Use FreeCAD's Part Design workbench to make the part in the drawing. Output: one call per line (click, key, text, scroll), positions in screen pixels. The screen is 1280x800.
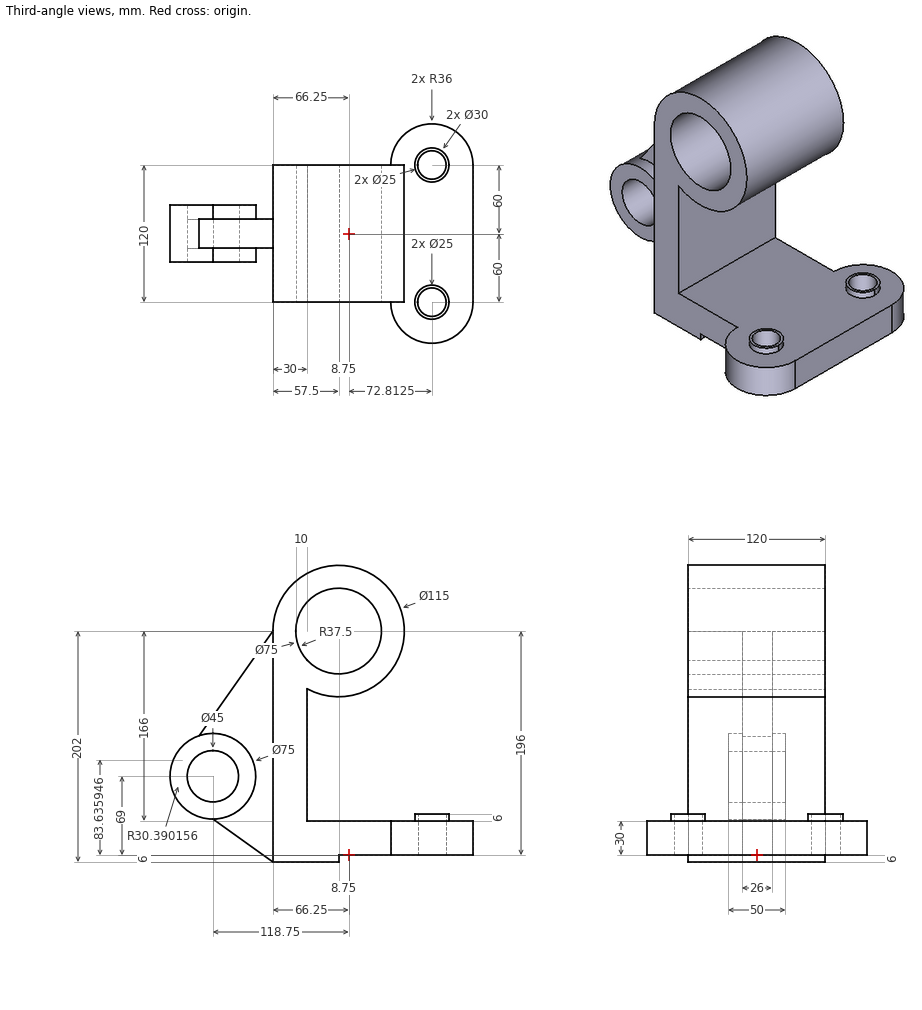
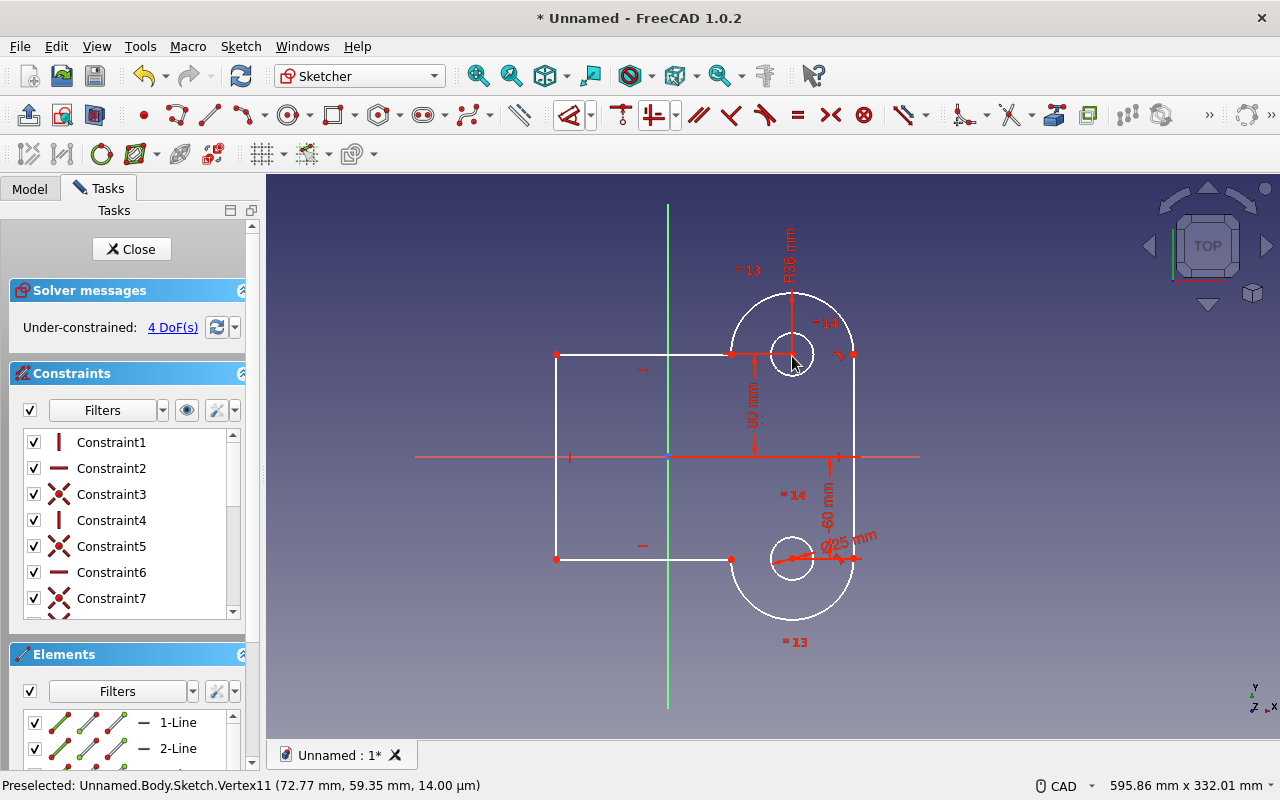
click(556, 416)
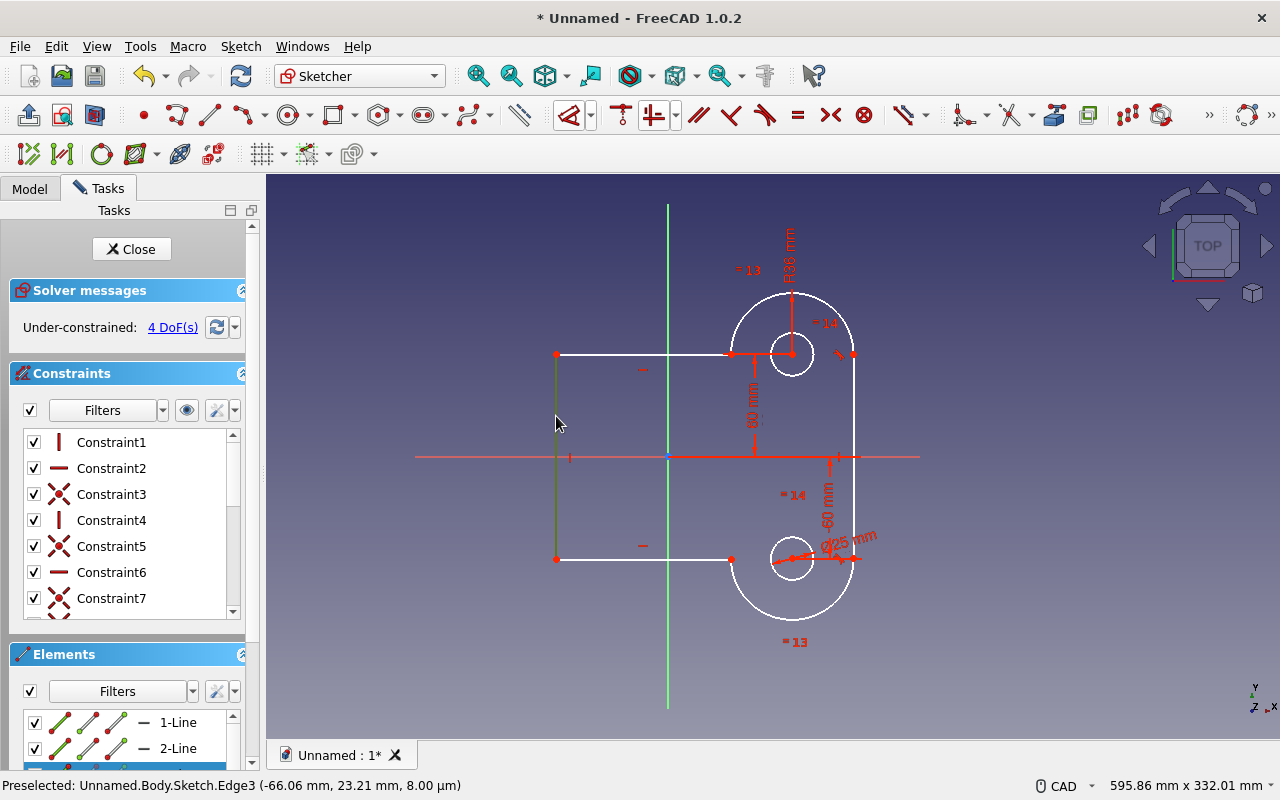
key(i)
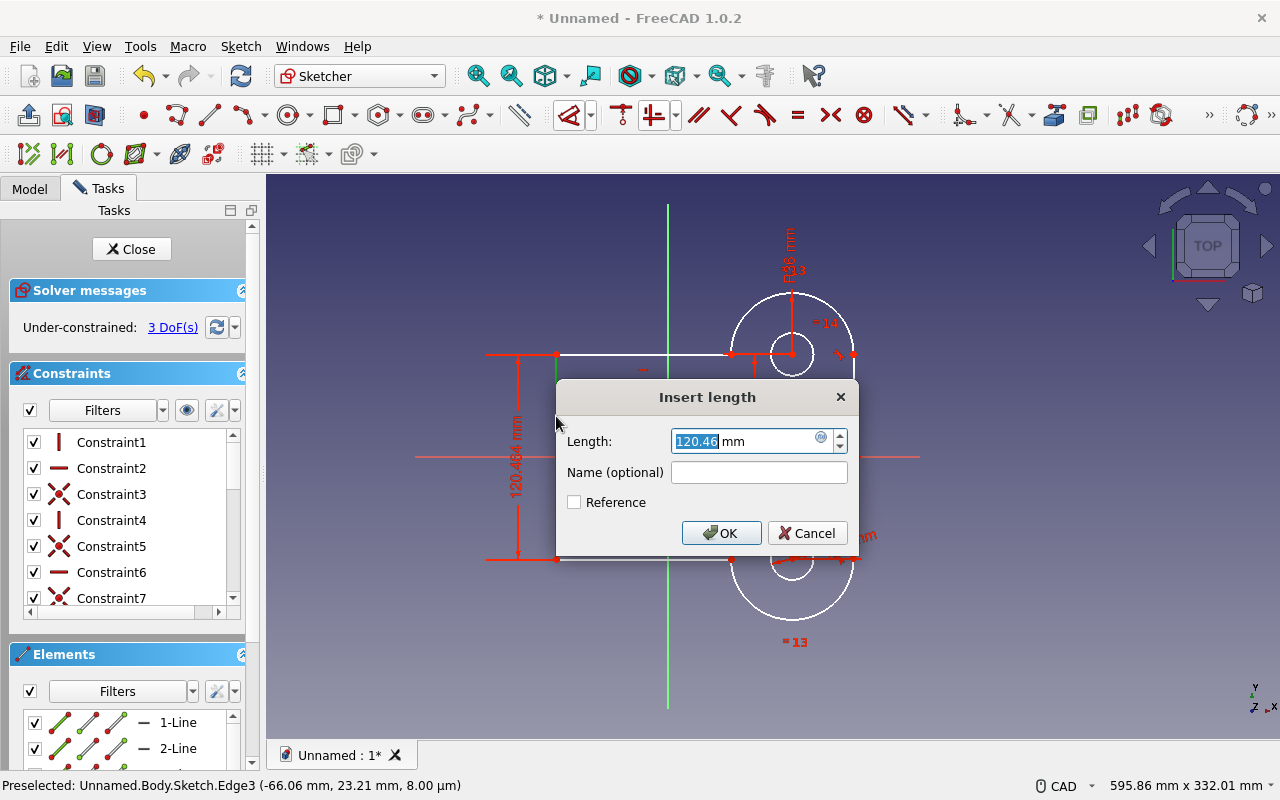
text(120)
key(Return)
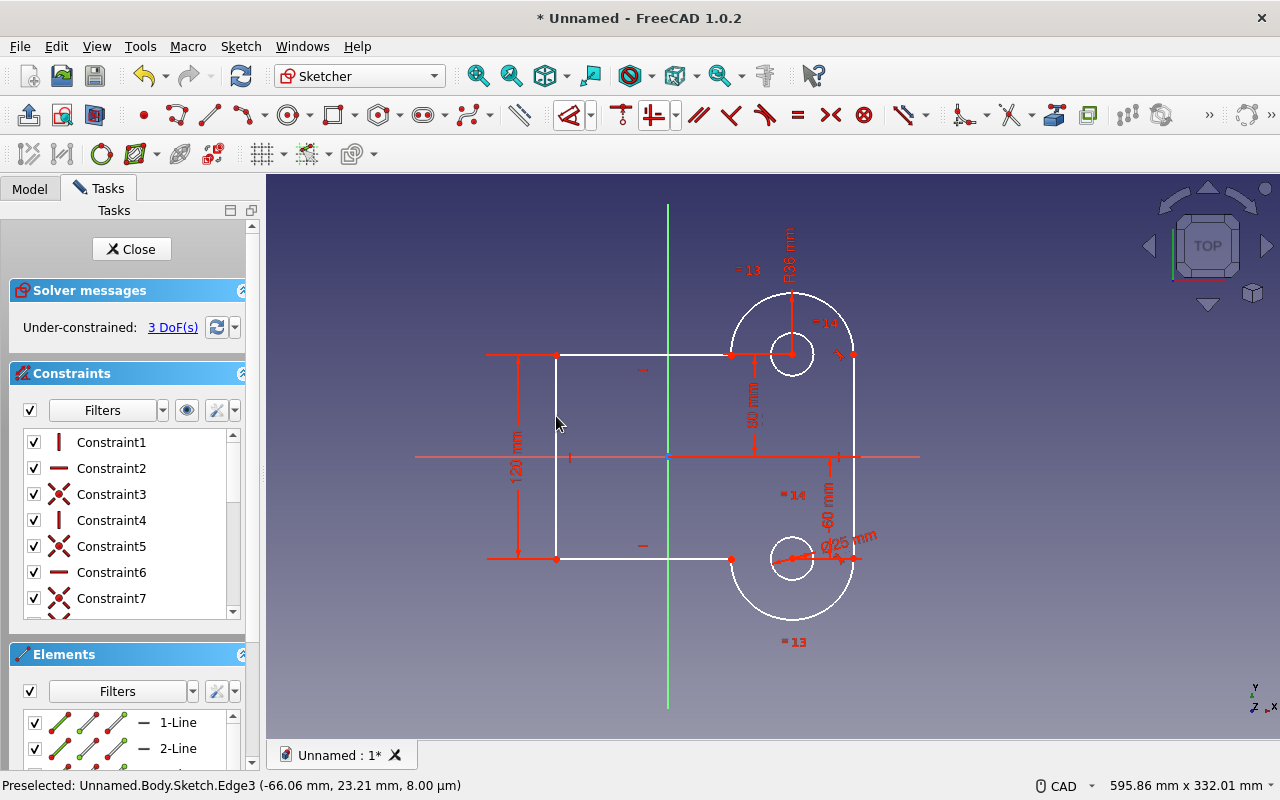
click(731, 355)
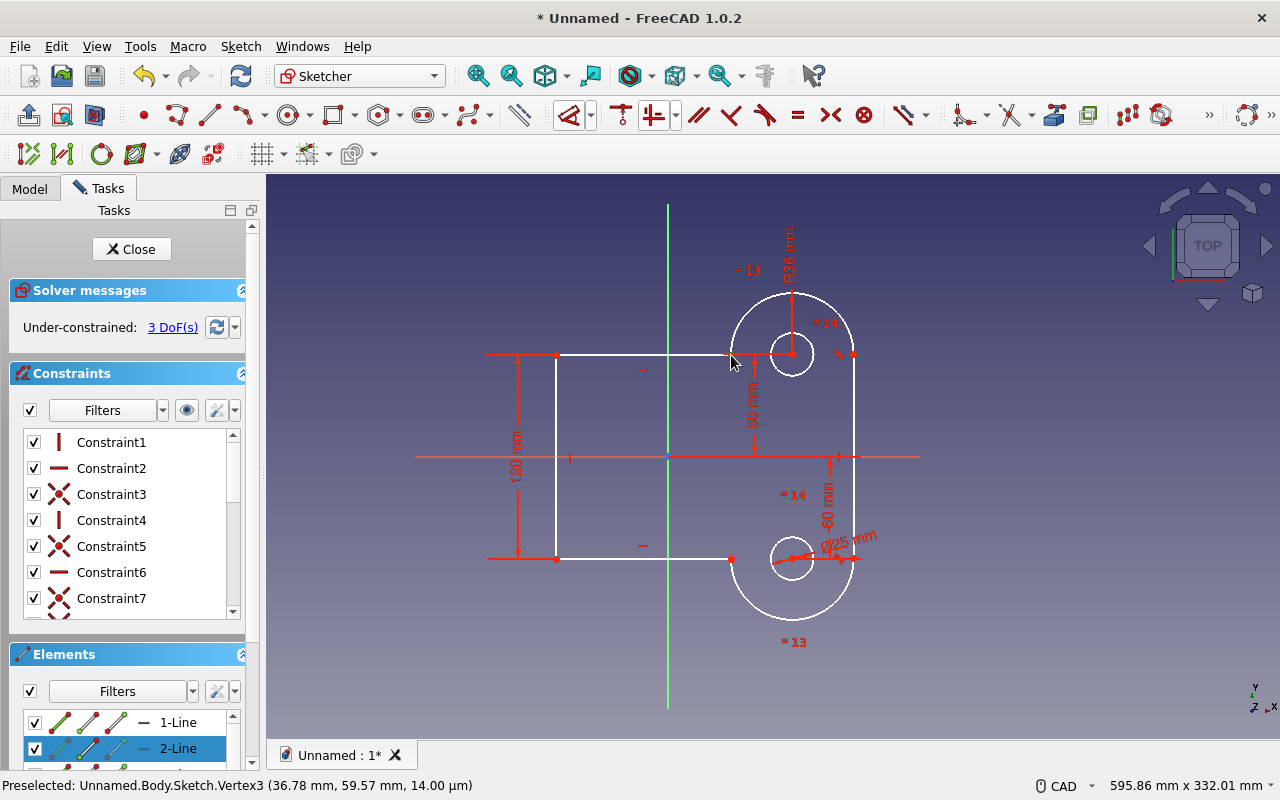
key(i)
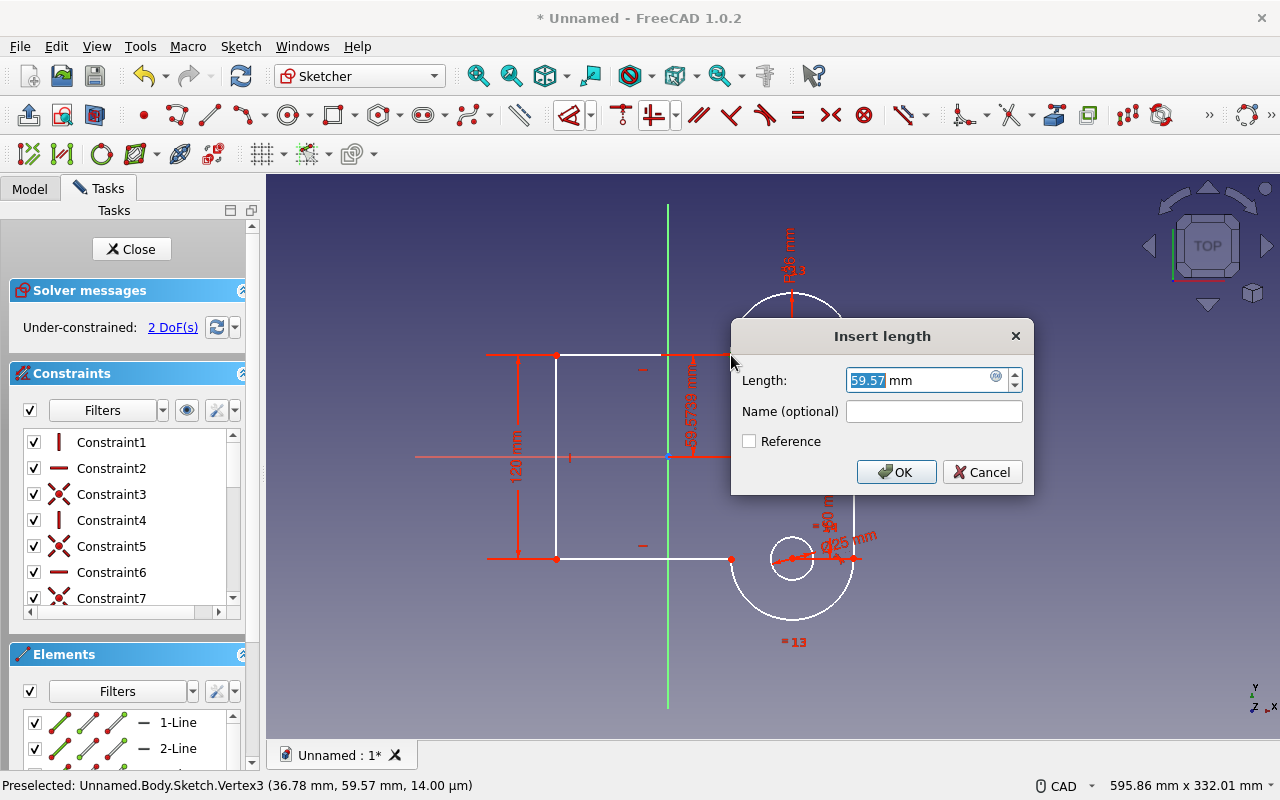
text(60)
key(Return)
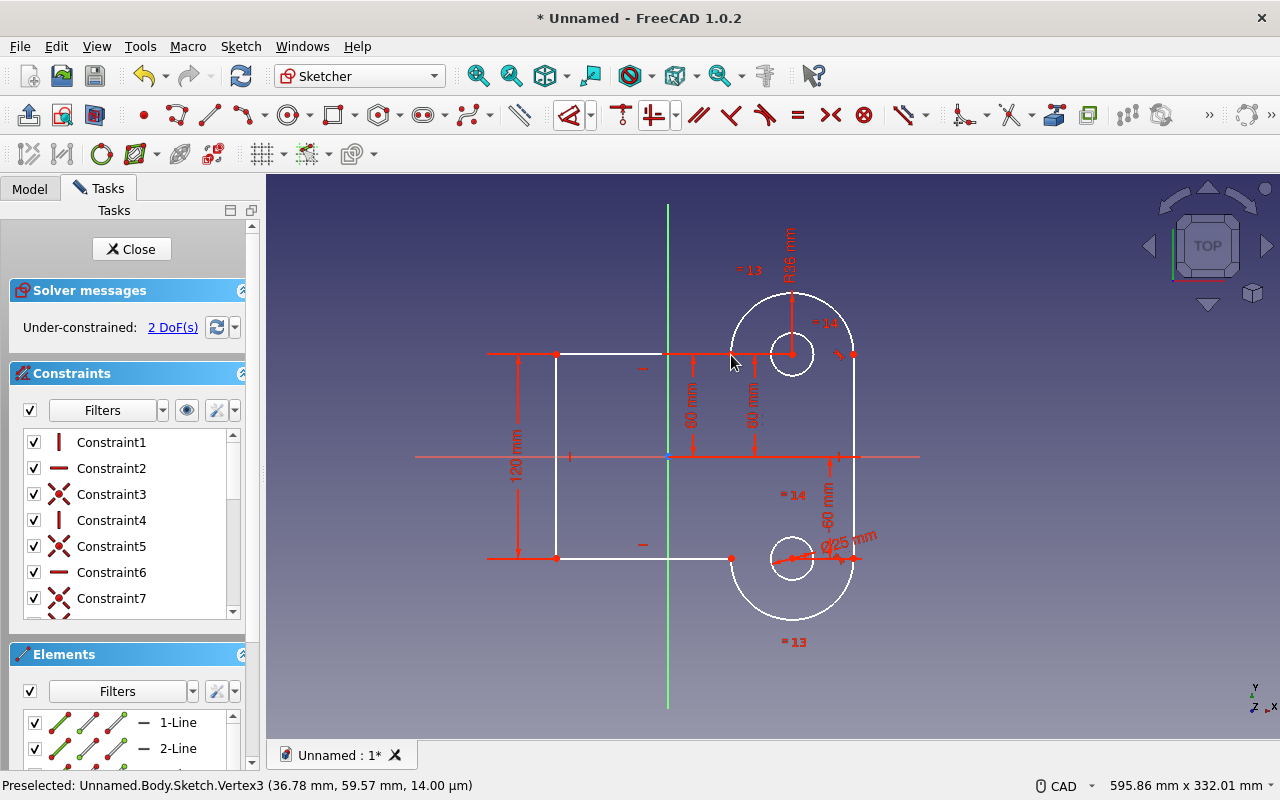
click(556, 354)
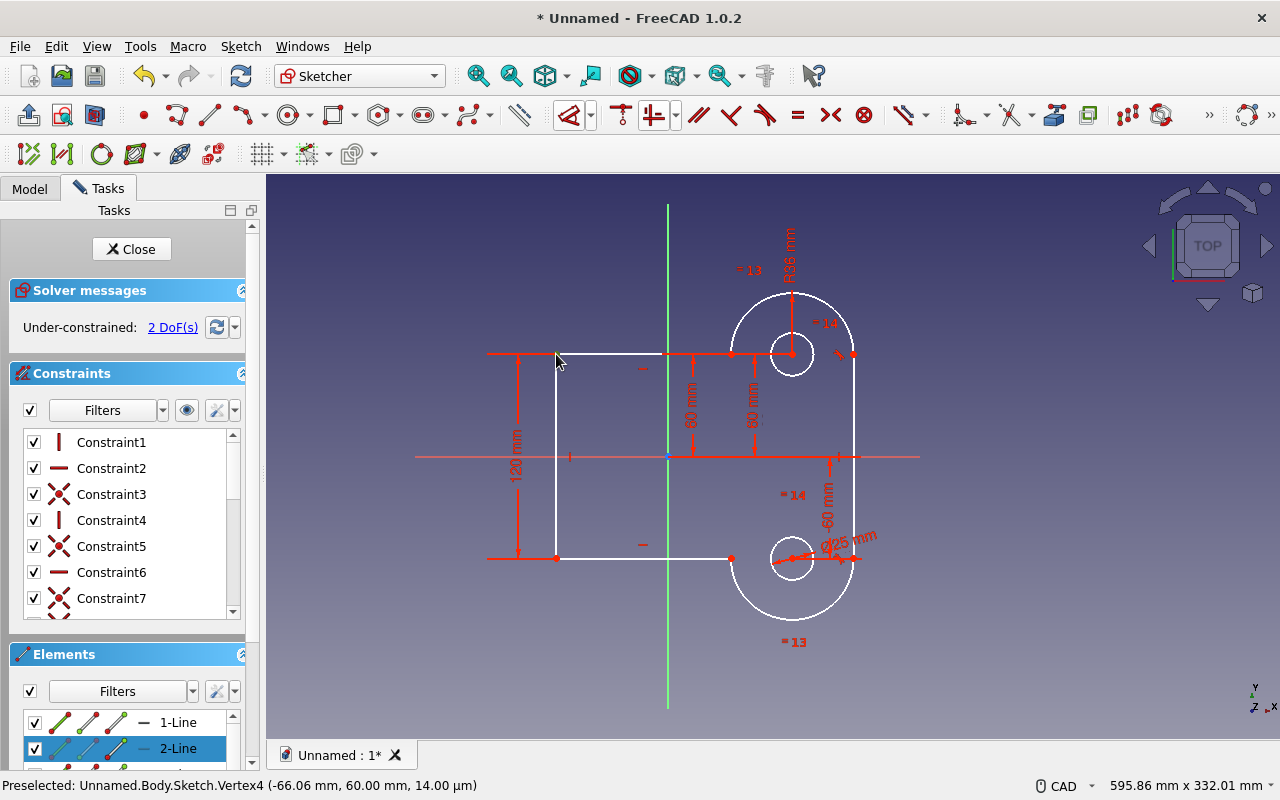
key(l)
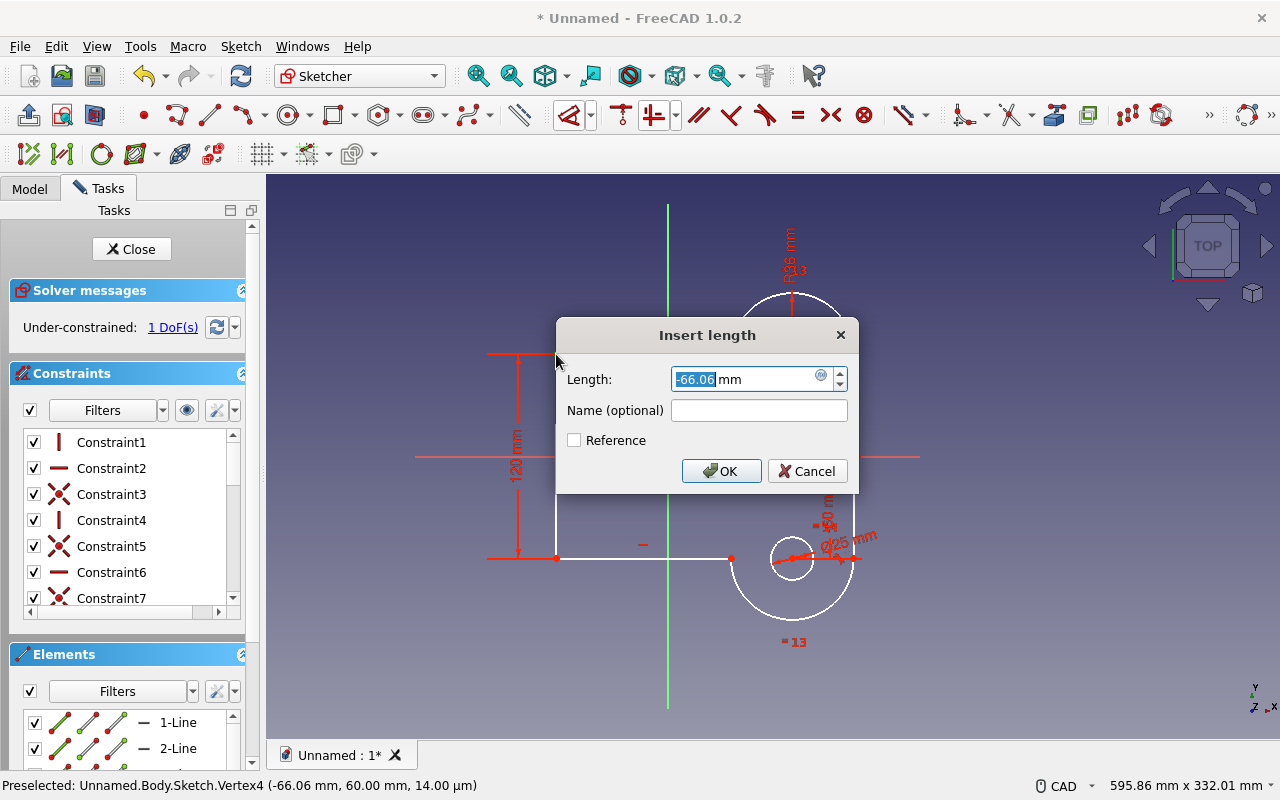
text(-66.25)
key(Return)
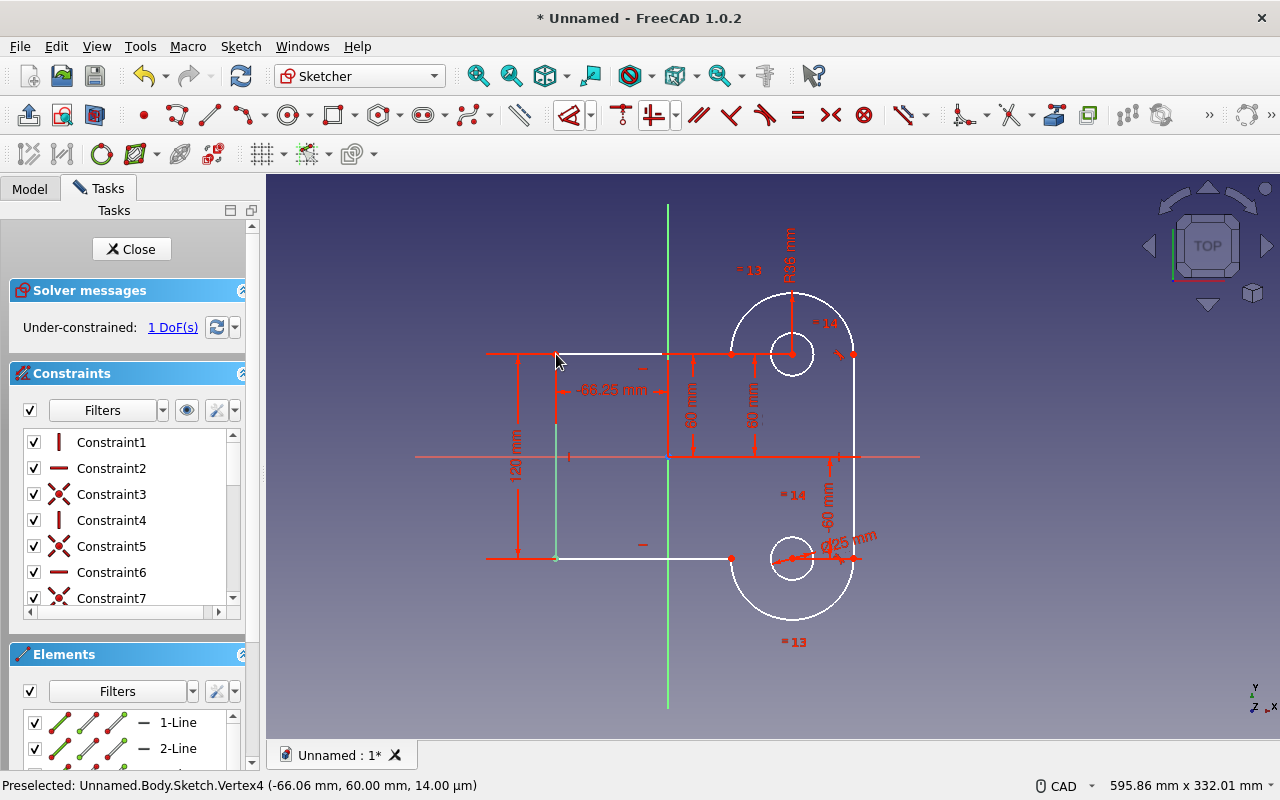
click(792, 559)